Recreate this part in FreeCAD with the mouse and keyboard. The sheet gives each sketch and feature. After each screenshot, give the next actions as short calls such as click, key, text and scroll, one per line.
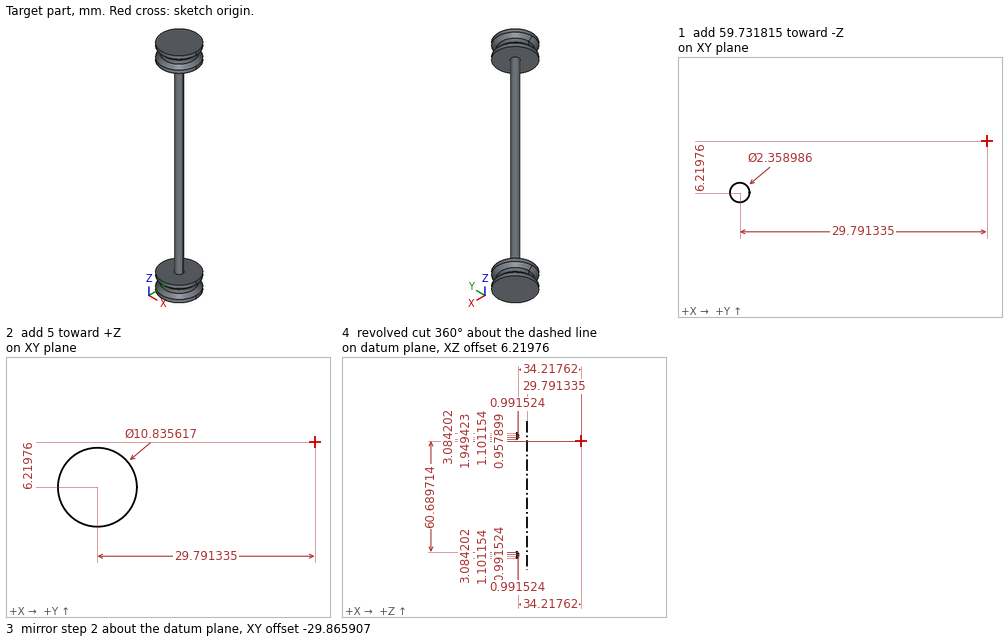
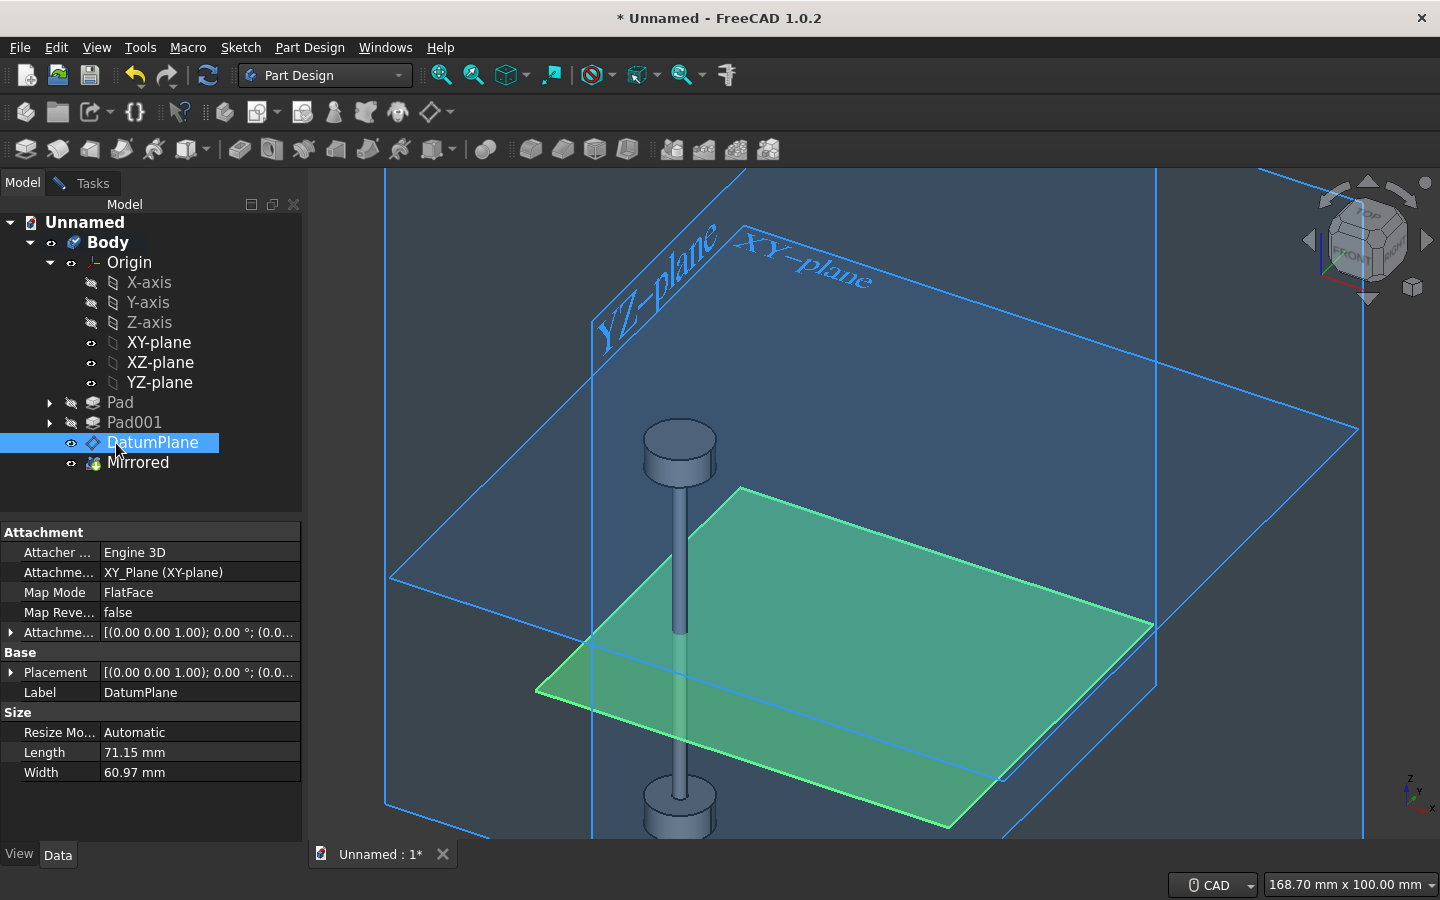
click(84, 182)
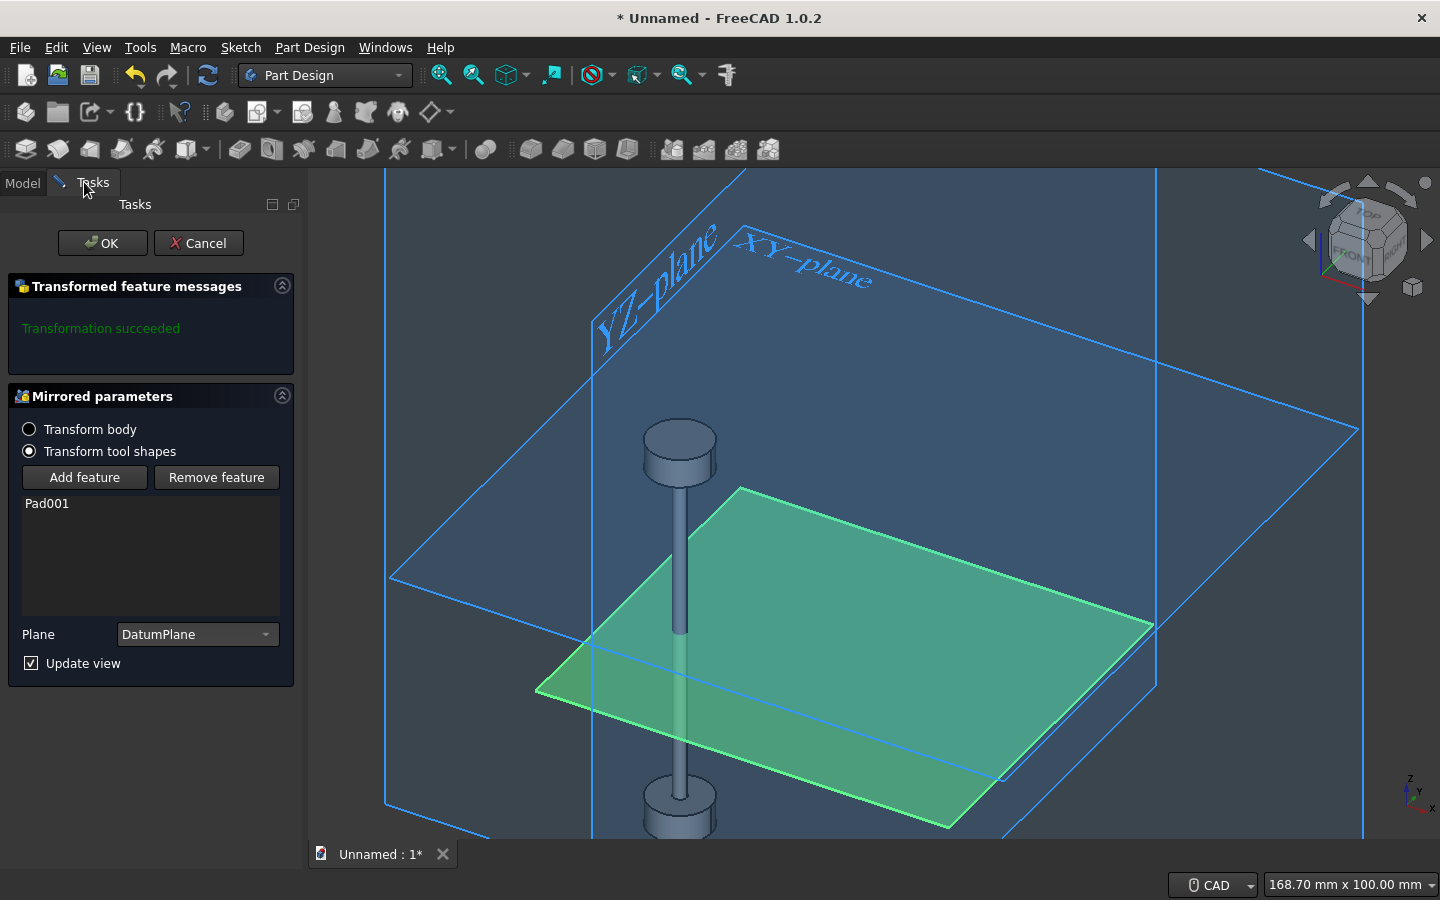
click(103, 243)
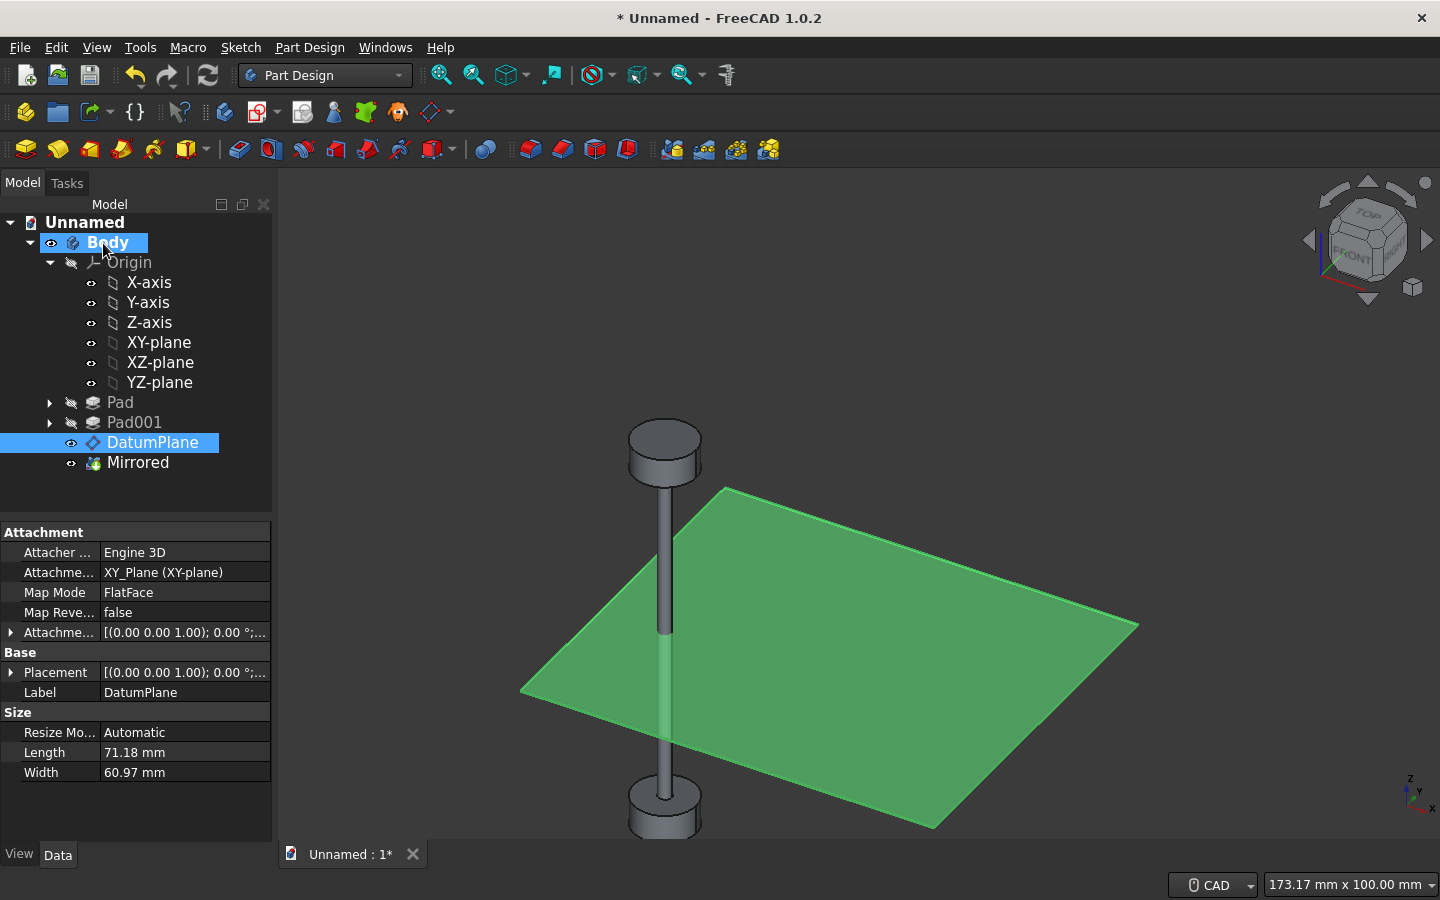
click(116, 443)
key(space)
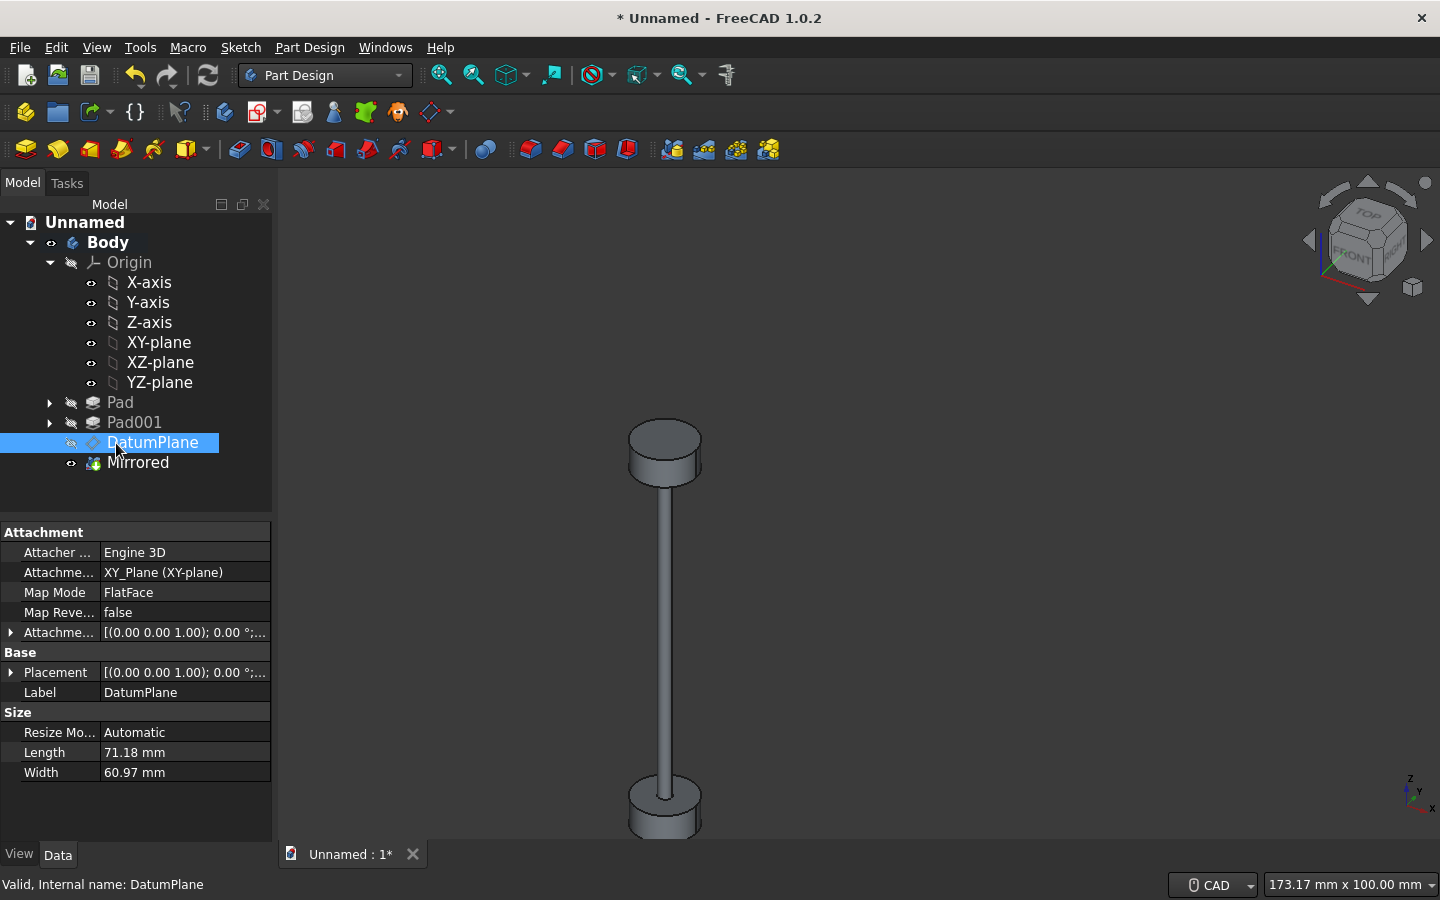
click(442, 76)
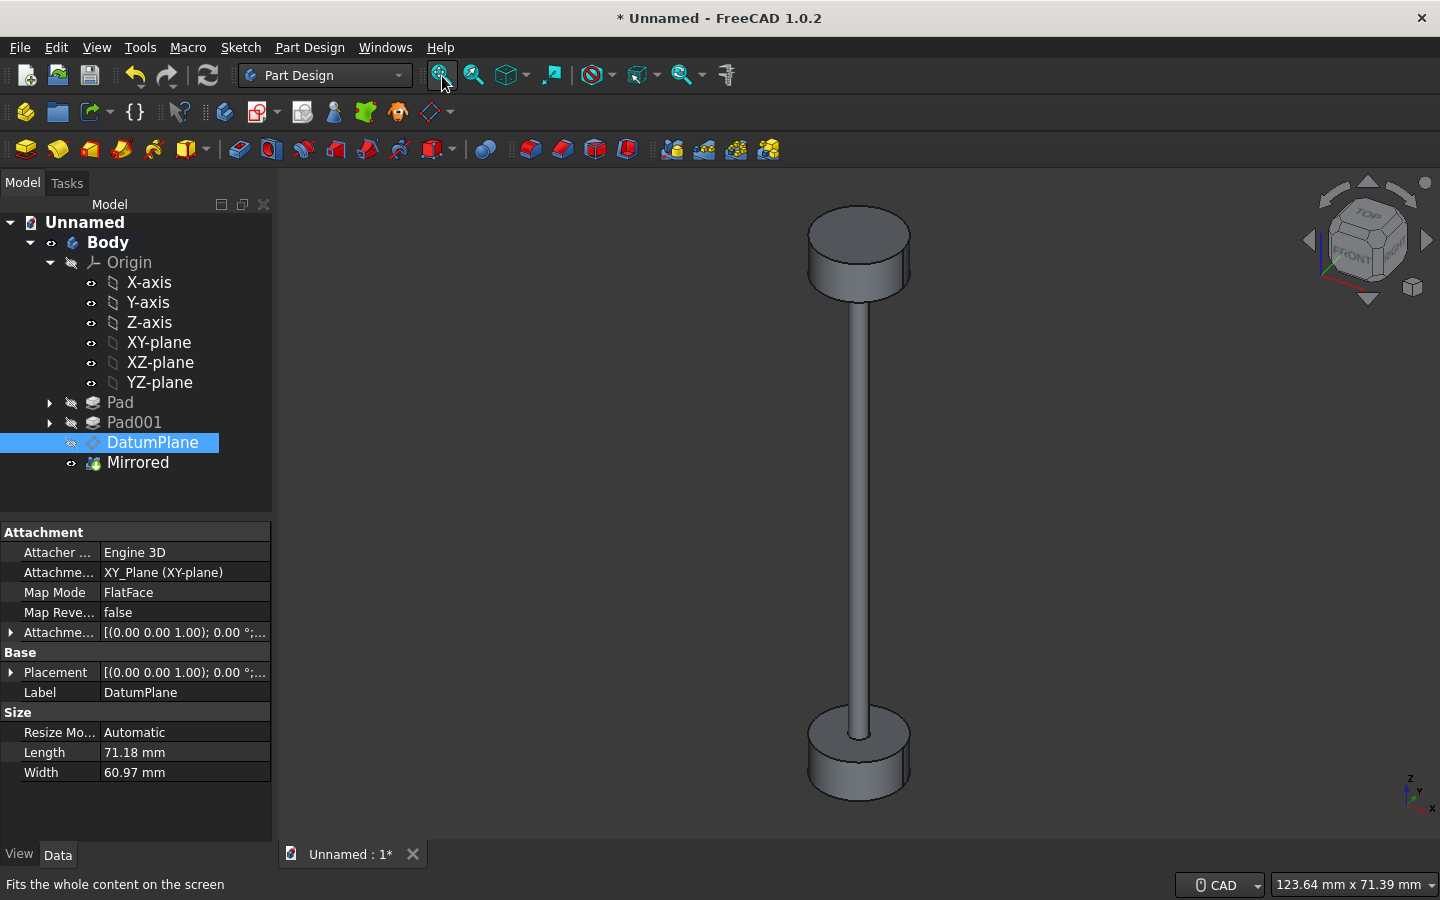
click(136, 363)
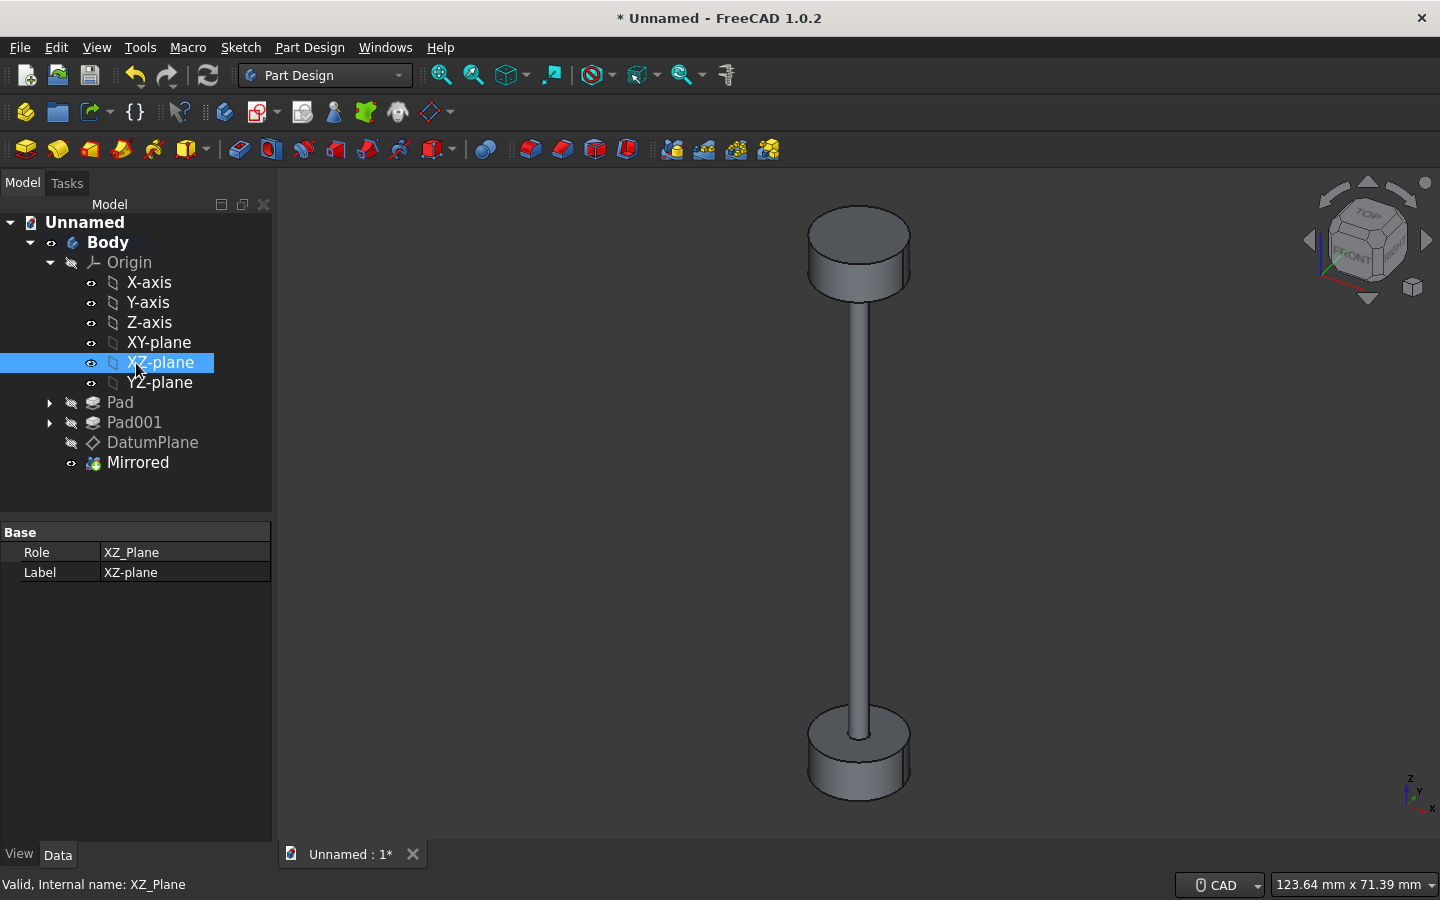
click(430, 112)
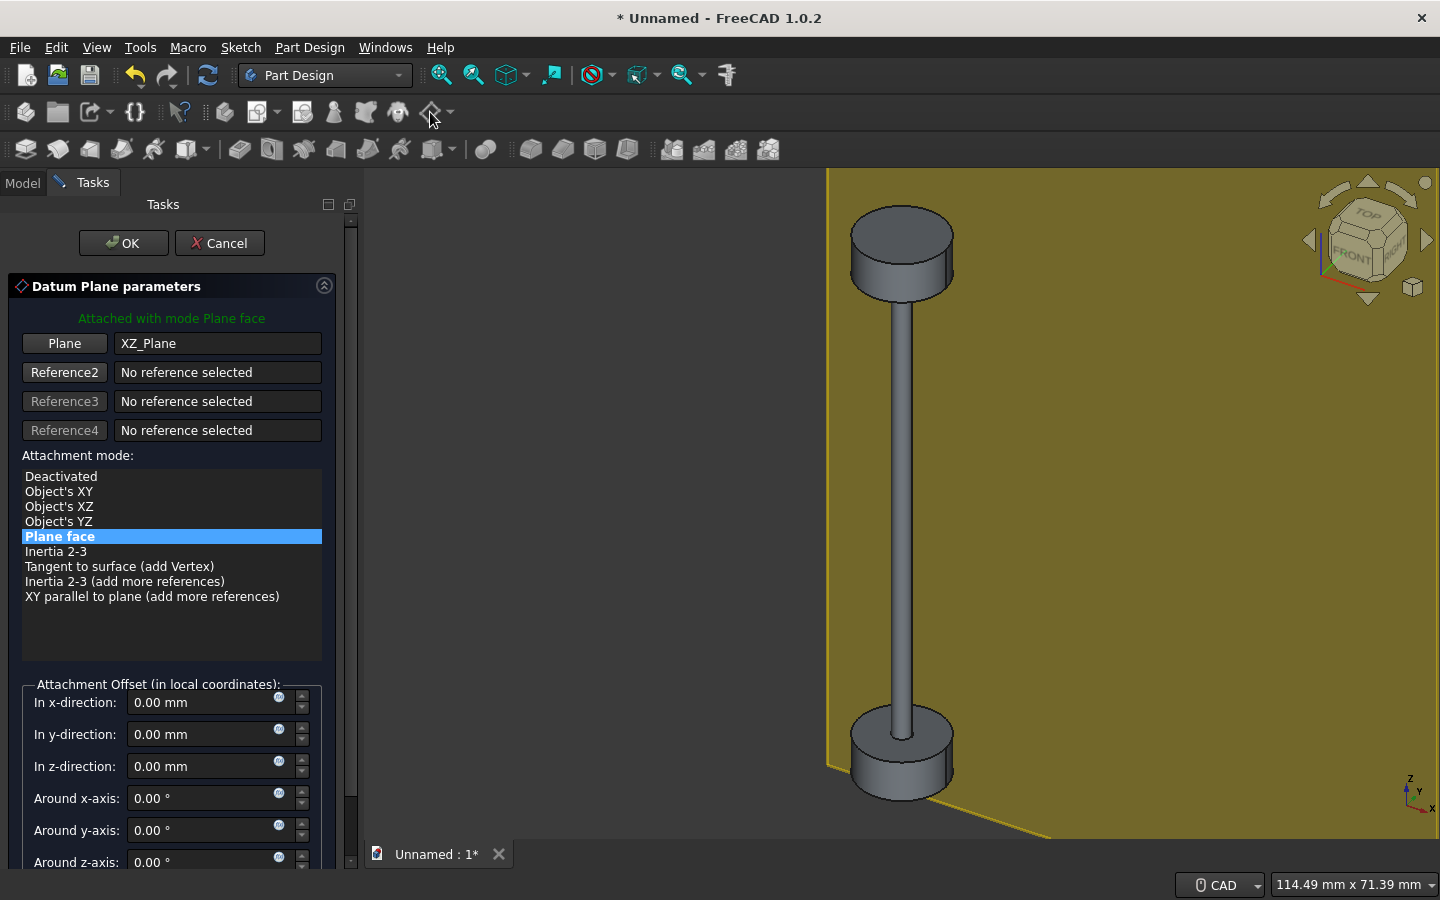
triple_click(210, 766)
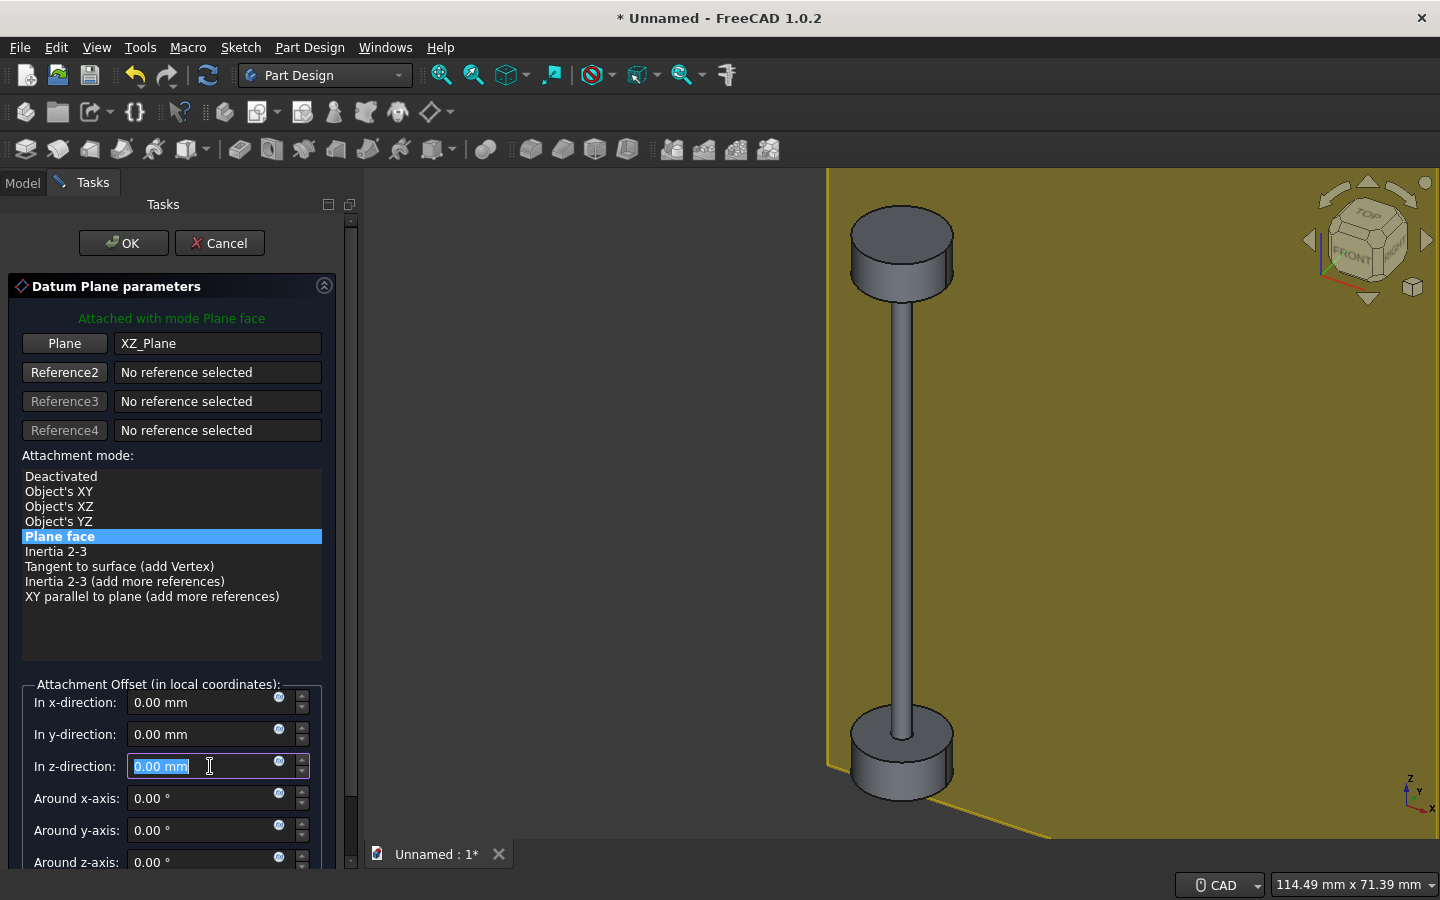
text(6.21976)
key(Tab)